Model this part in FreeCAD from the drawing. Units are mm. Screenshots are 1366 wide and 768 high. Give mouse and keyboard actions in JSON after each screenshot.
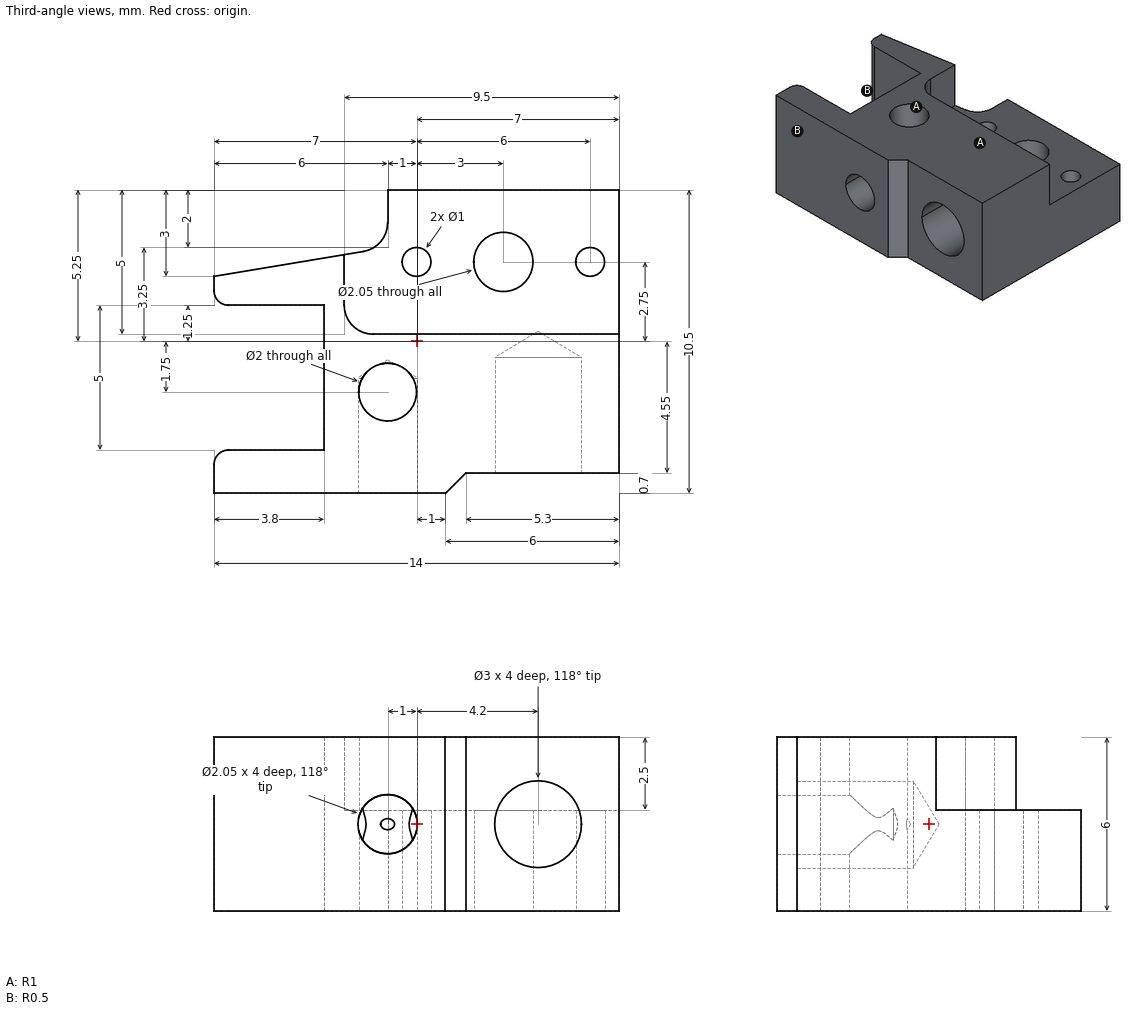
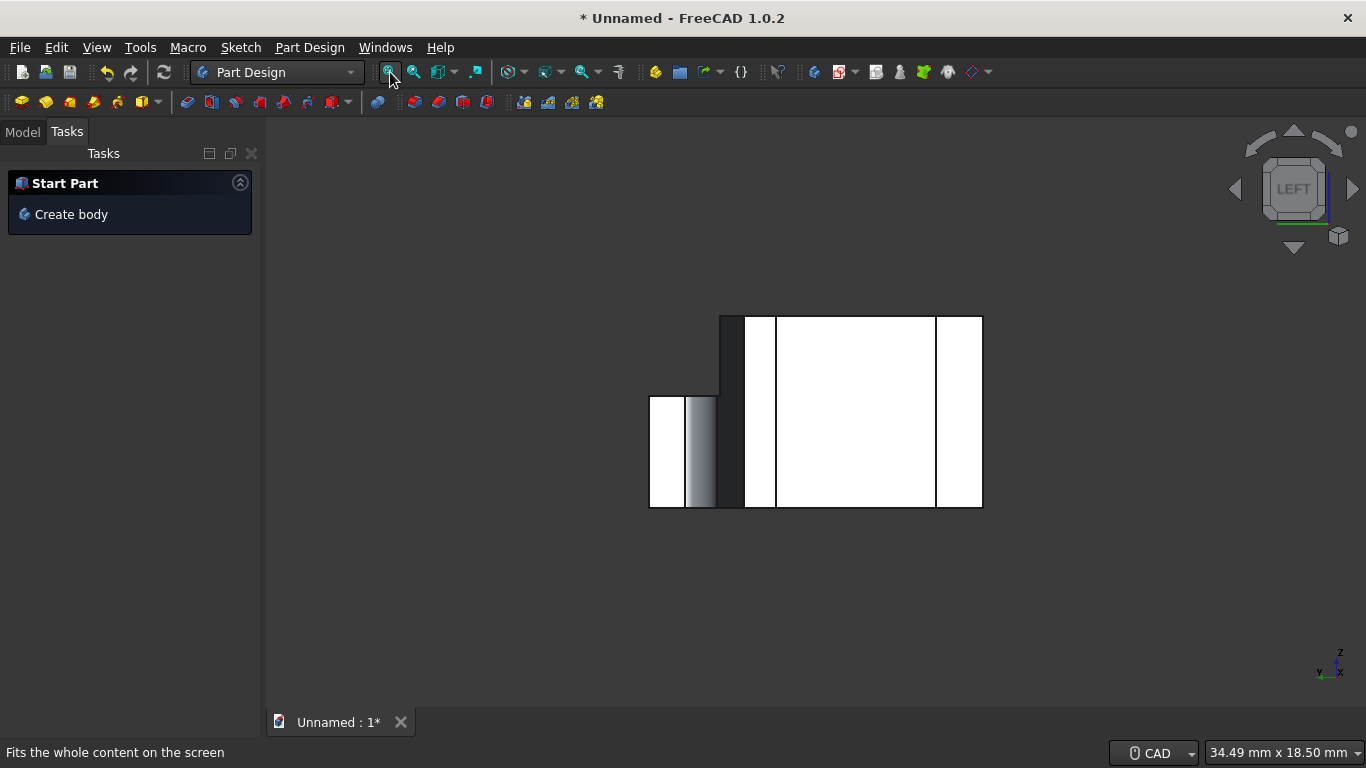
{"action": "left_click", "coordinate": [936, 411]}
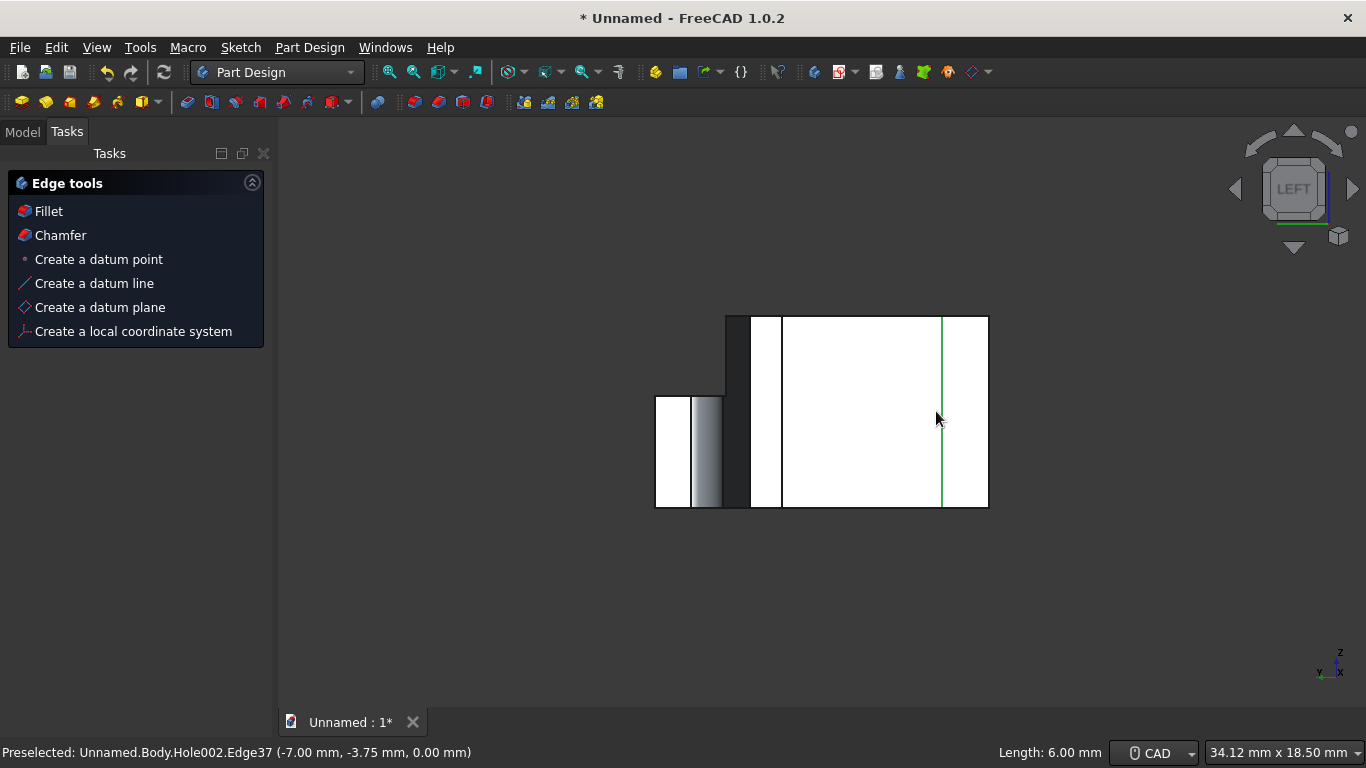
{"action": "left_click", "coordinate": [782, 411], "text": "ctrl"}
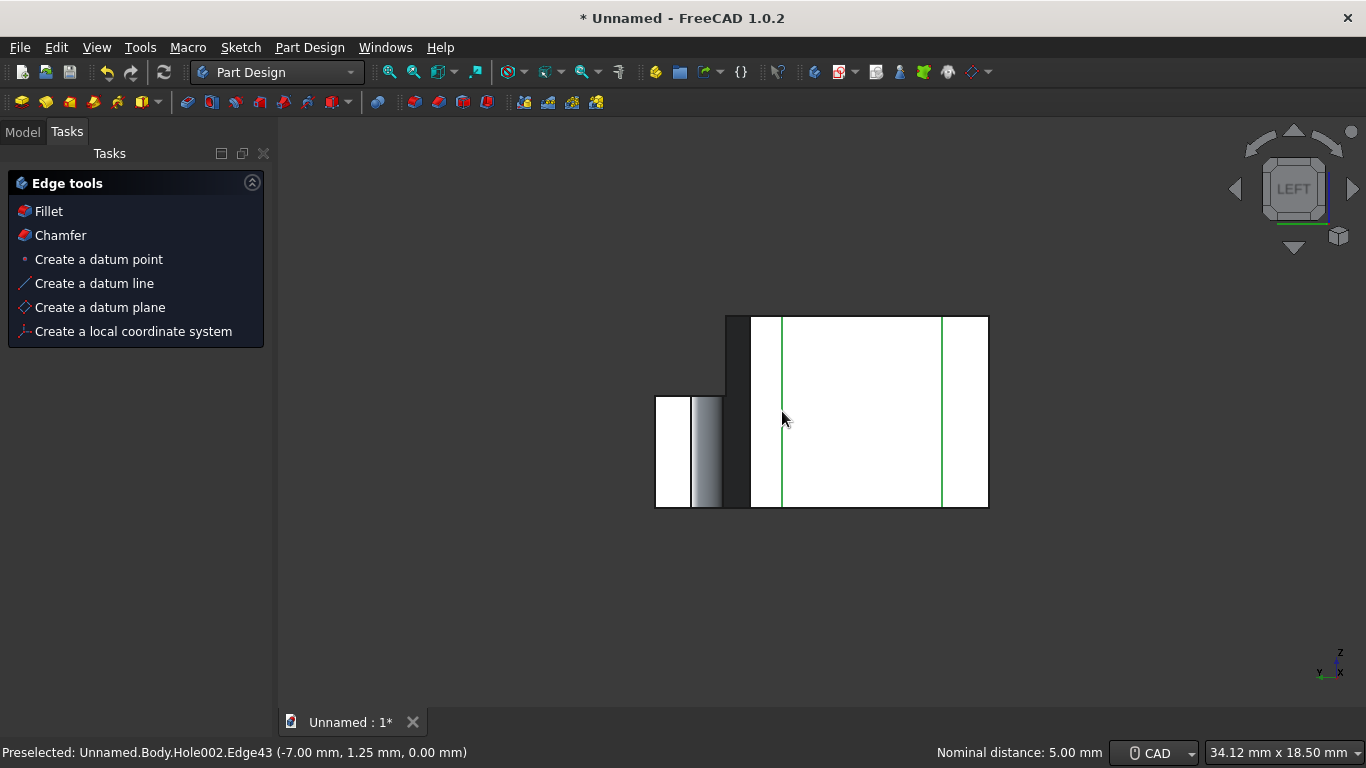
{"action": "left_click", "coordinate": [416, 102]}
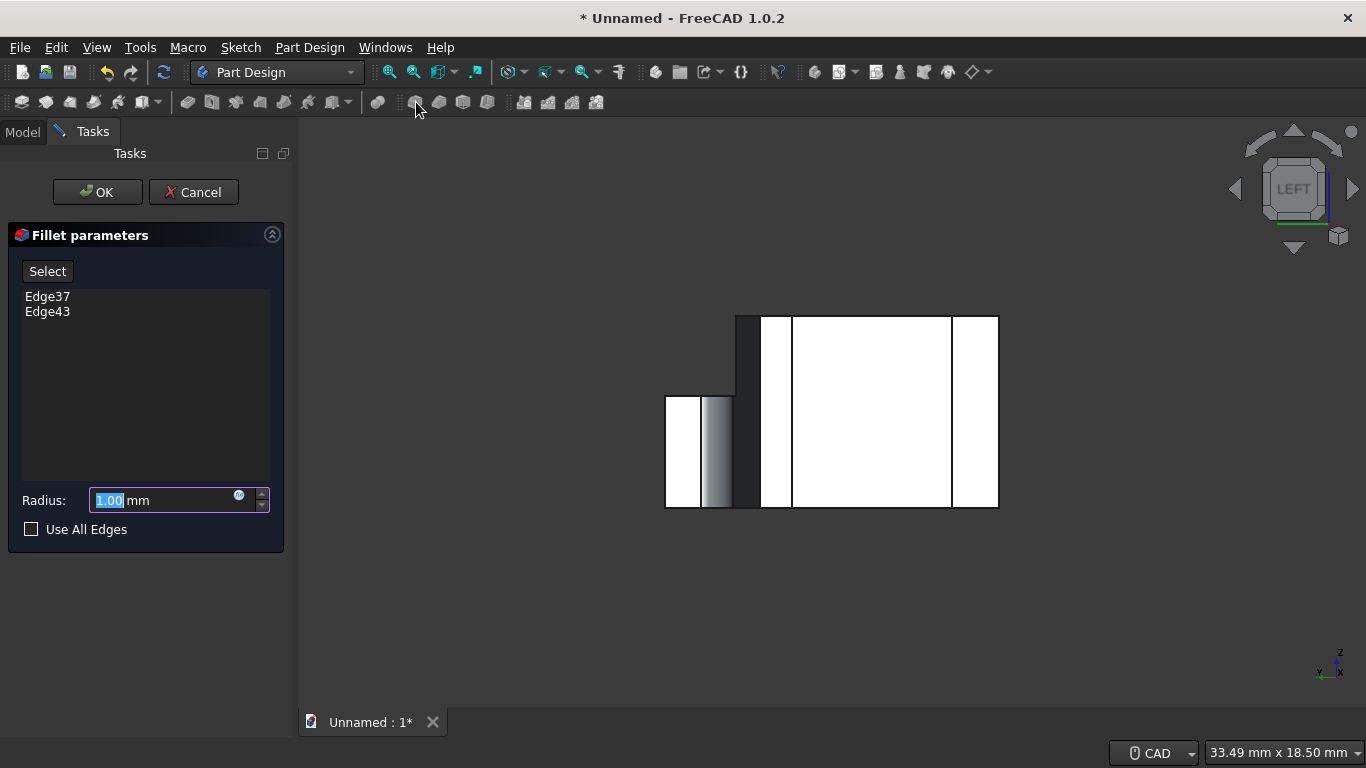
{"action": "type", "text": "0.5"}
{"action": "key", "text": "Tab"}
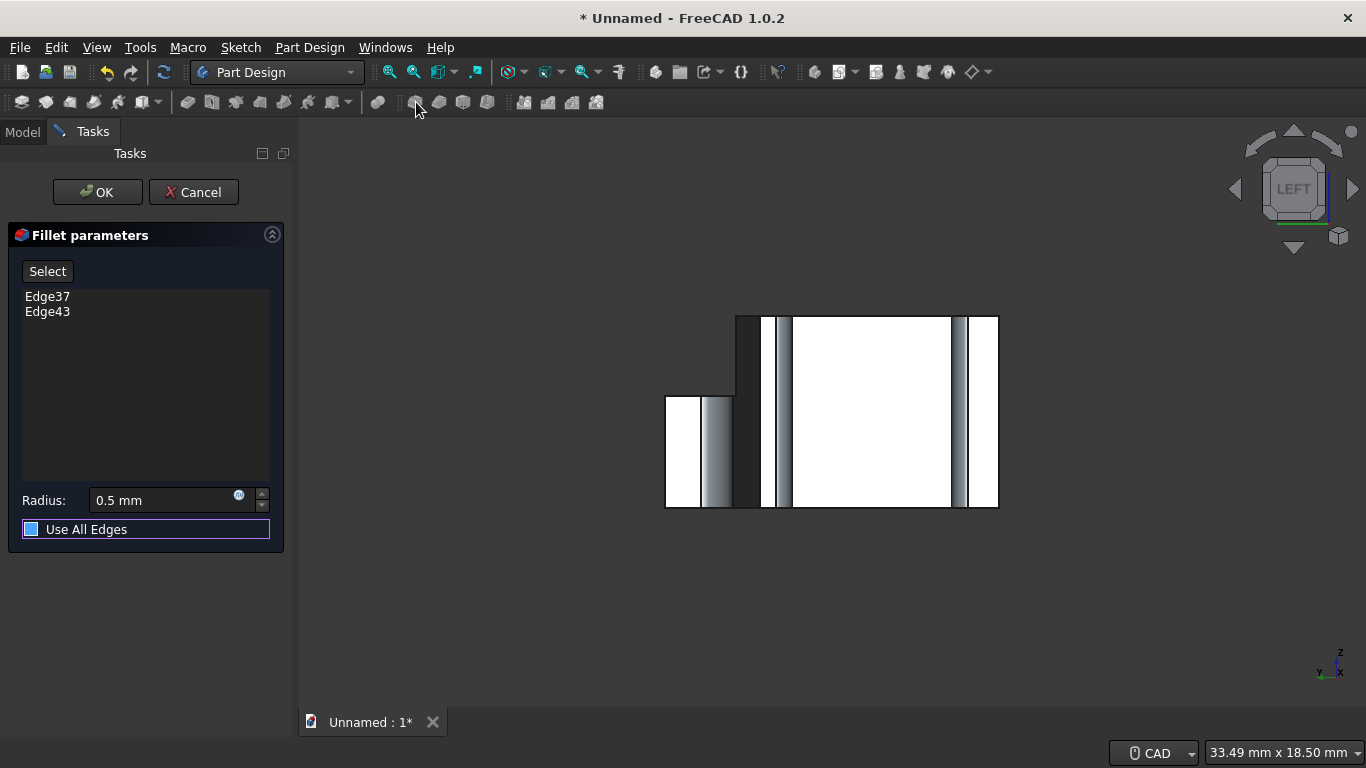
{"action": "left_click", "coordinate": [98, 192]}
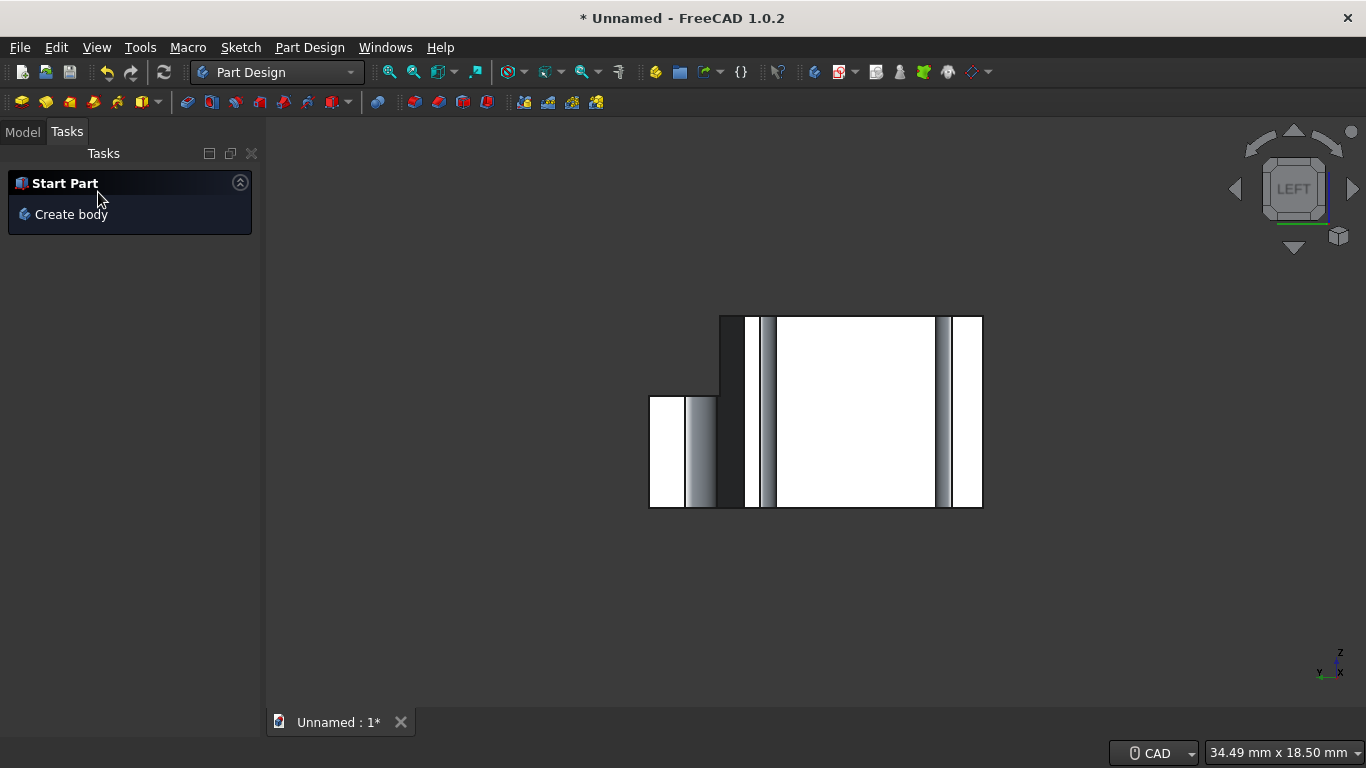
{"action": "left_click", "coordinate": [390, 72]}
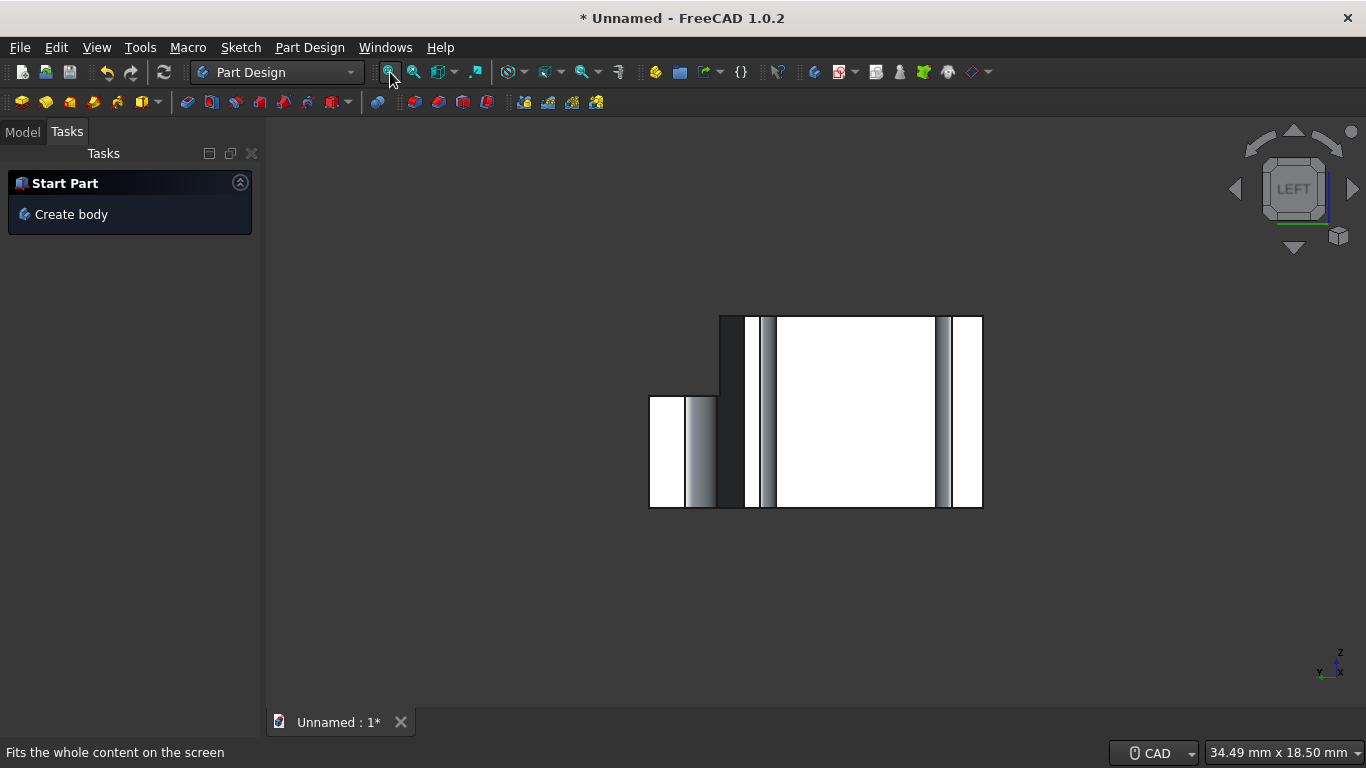
{"action": "key", "text": "0"}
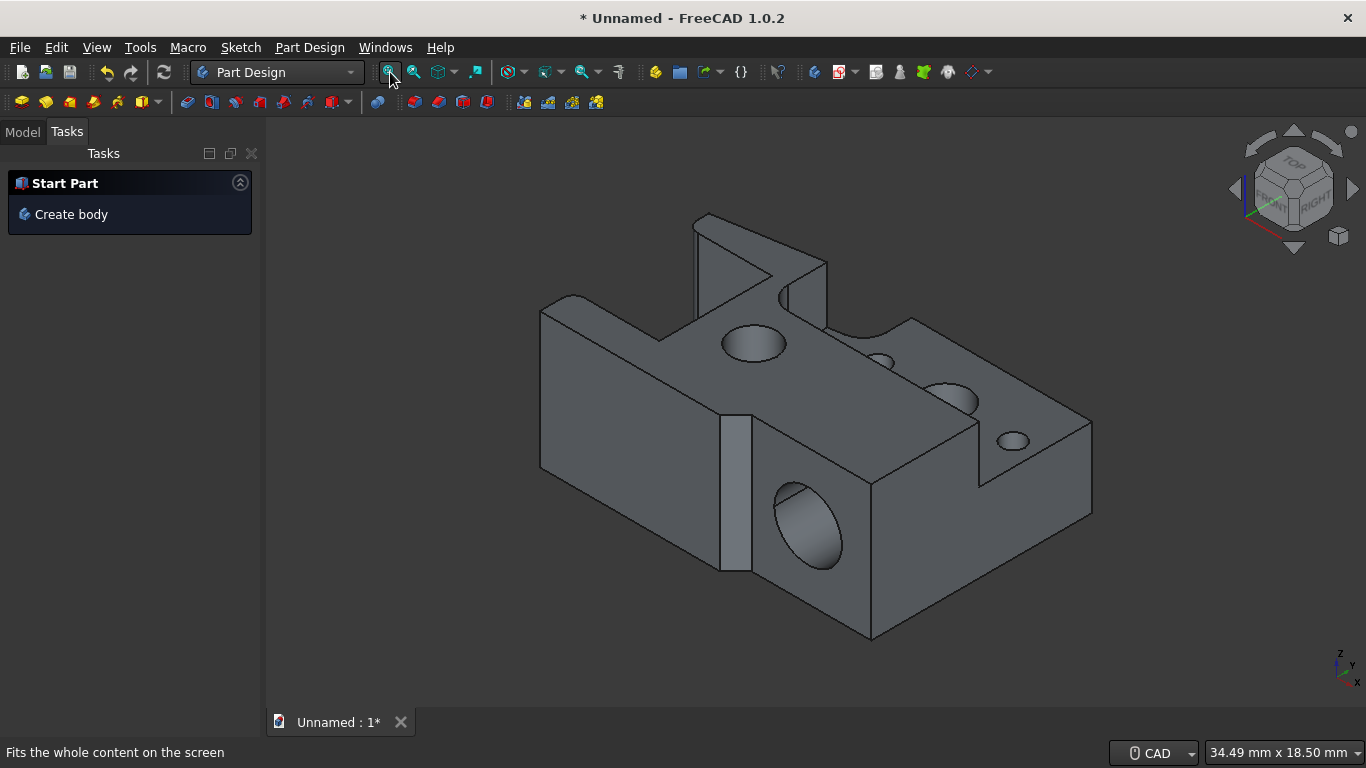
{"action": "left_click", "coordinate": [630, 440]}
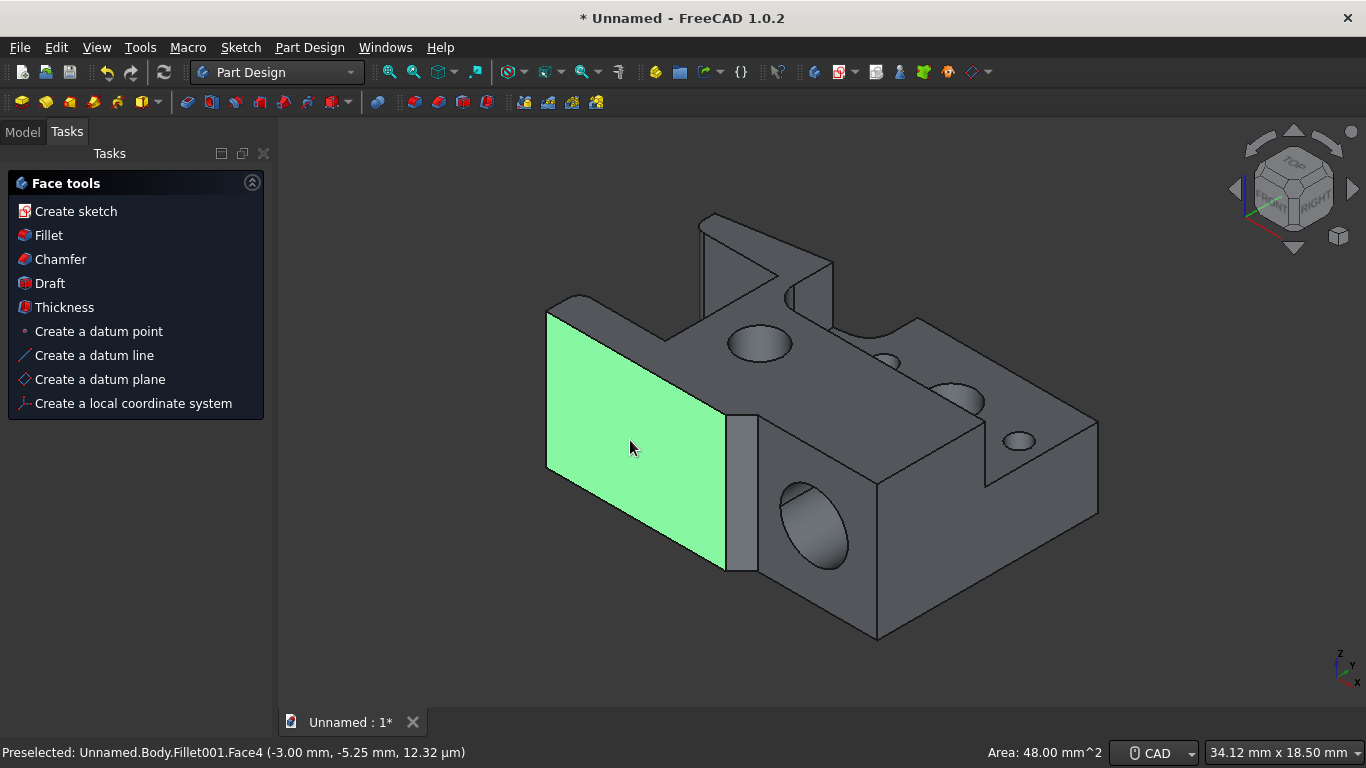
{"action": "left_click", "coordinate": [840, 72]}